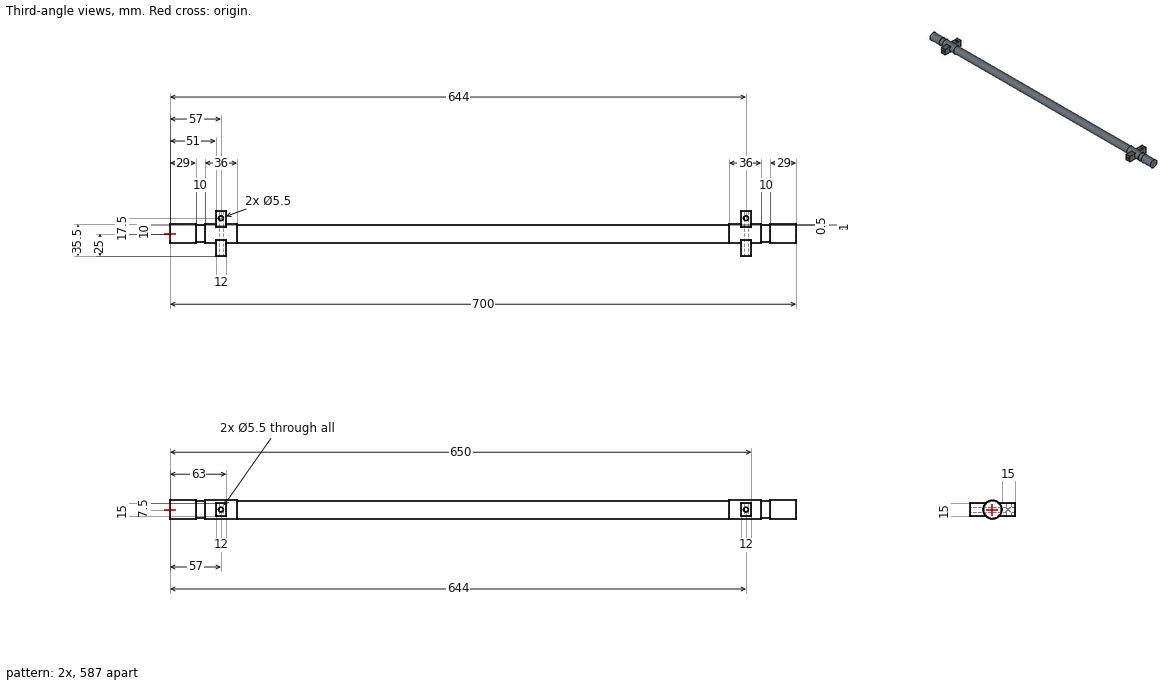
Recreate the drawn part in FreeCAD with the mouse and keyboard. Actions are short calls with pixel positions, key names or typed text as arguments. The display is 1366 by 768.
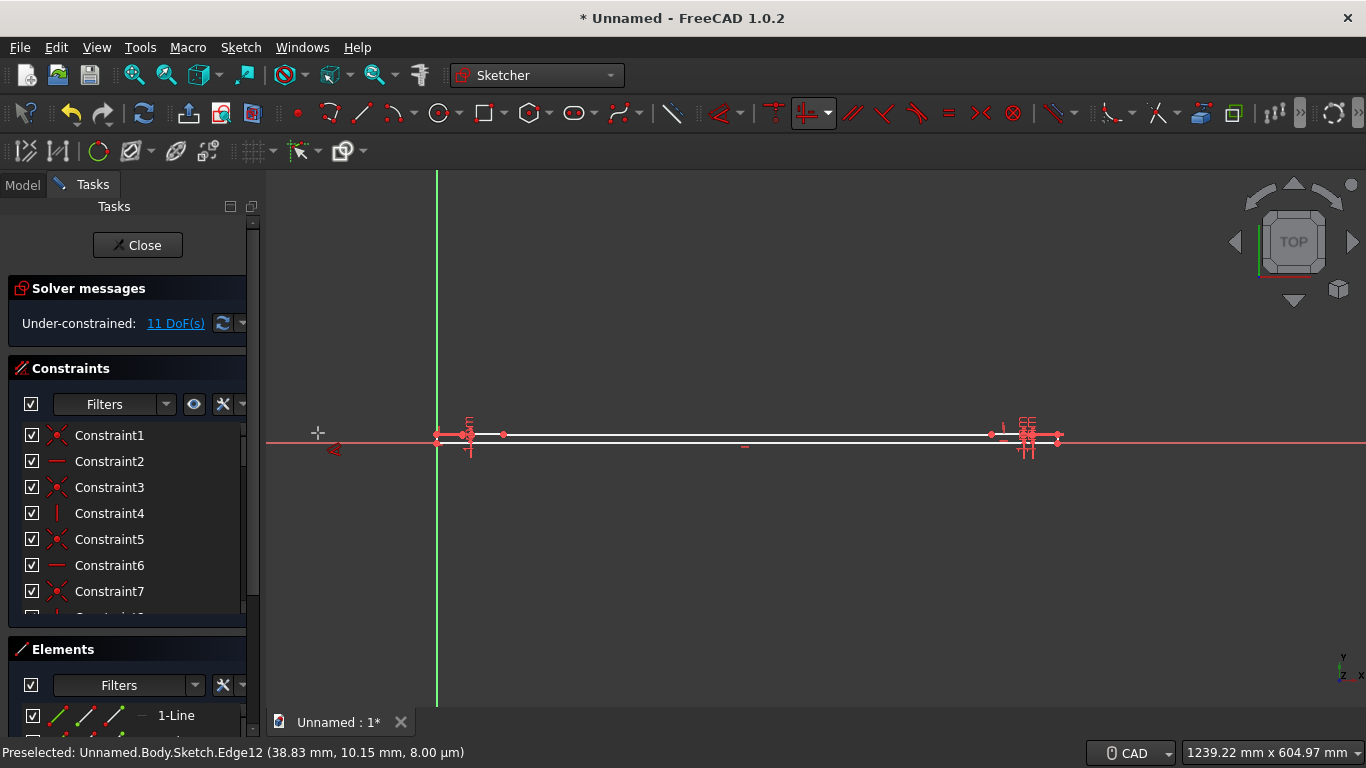
scroll(462, 435, up, 20)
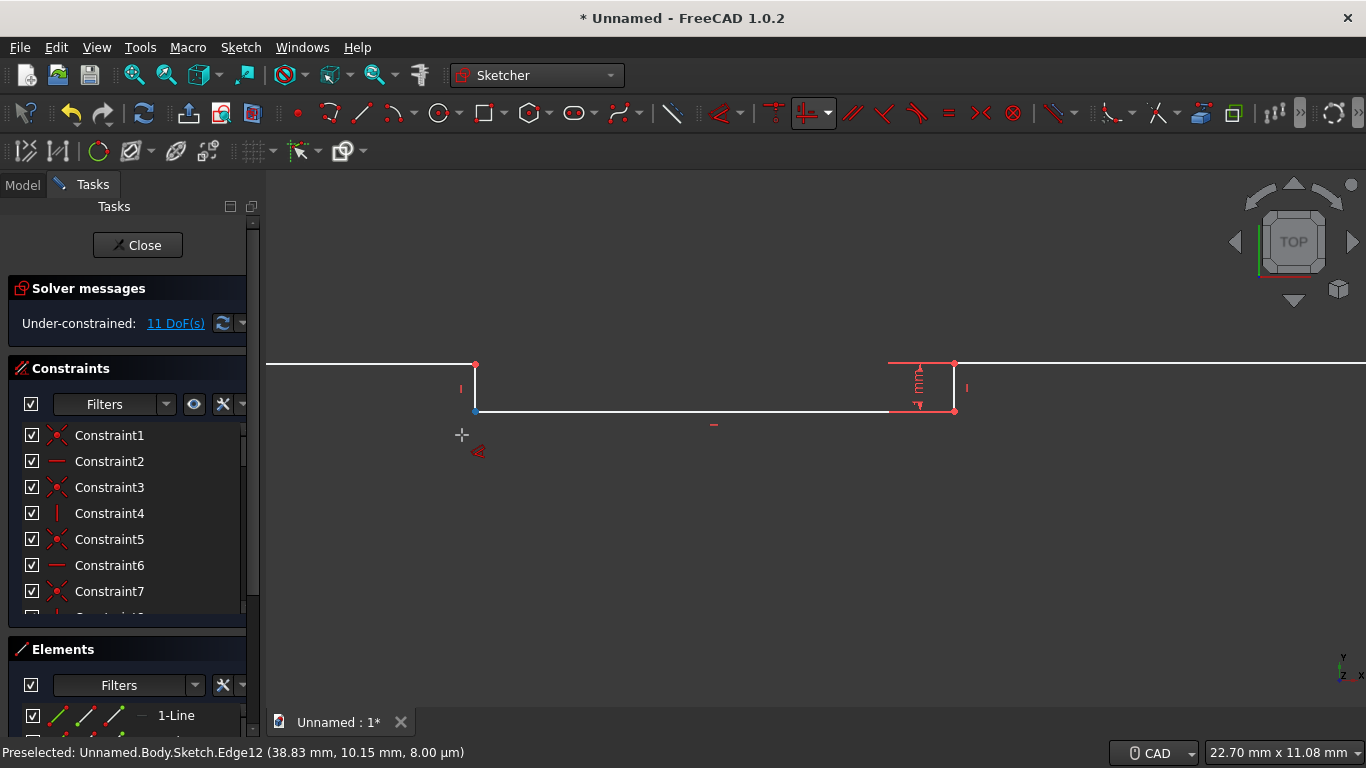
click(475, 397)
click(441, 388)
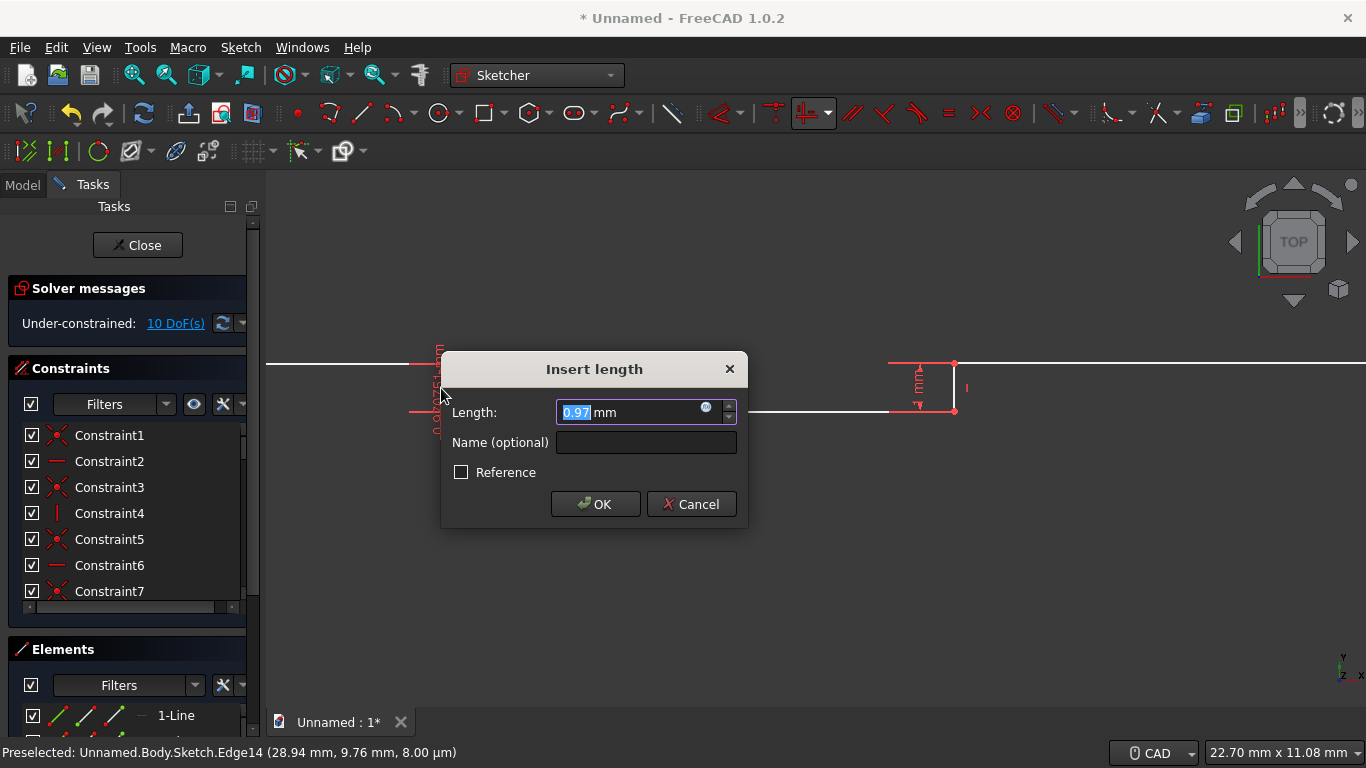
text(1)
key(Return)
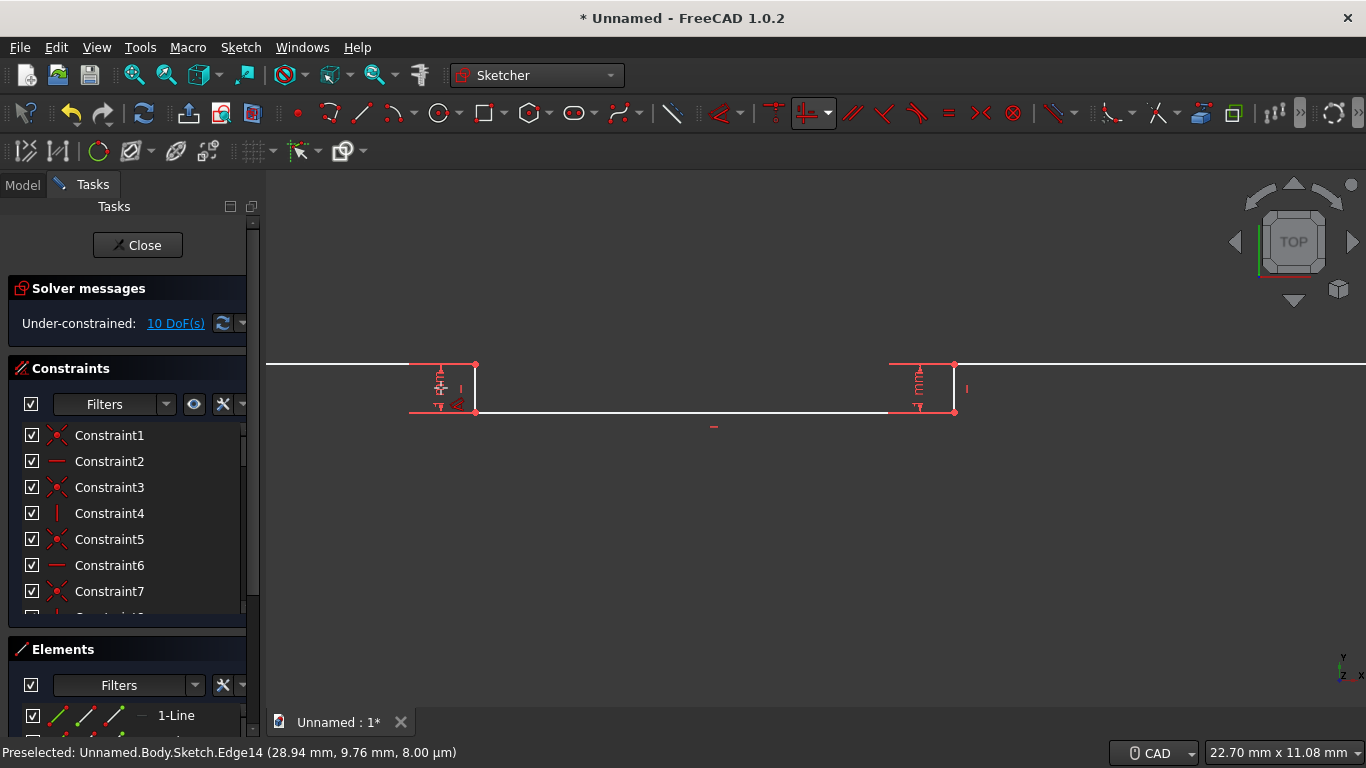
scroll(748, 438, down, 15)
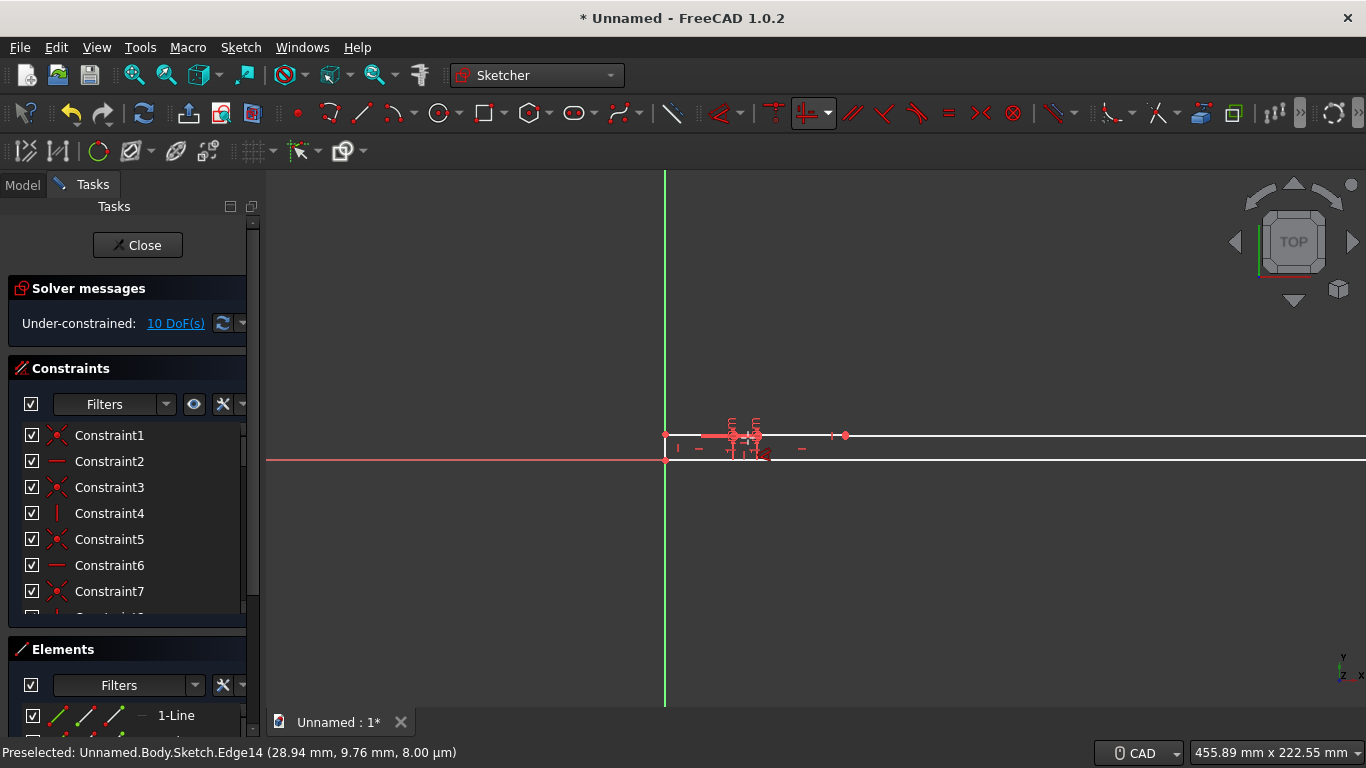
scroll(304, 433, down, 5)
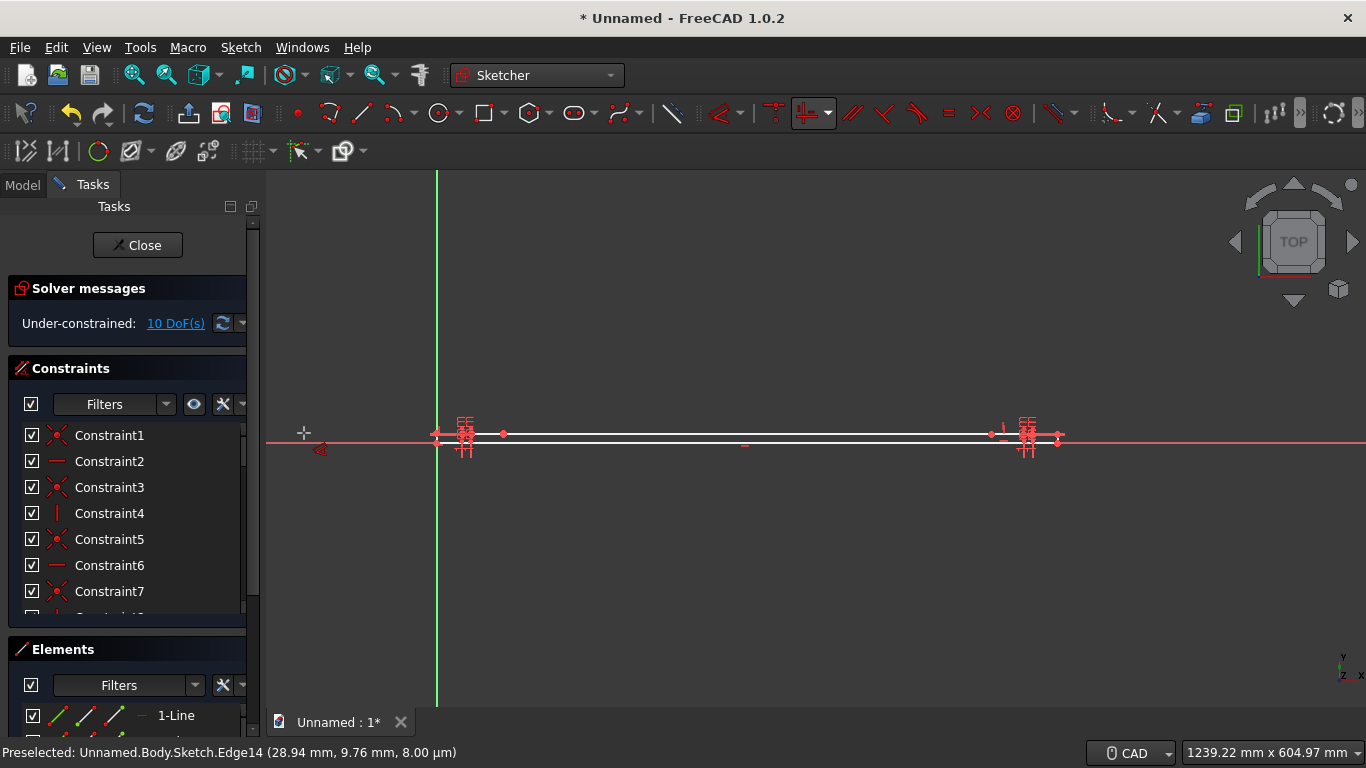
scroll(1050, 434, up, 3)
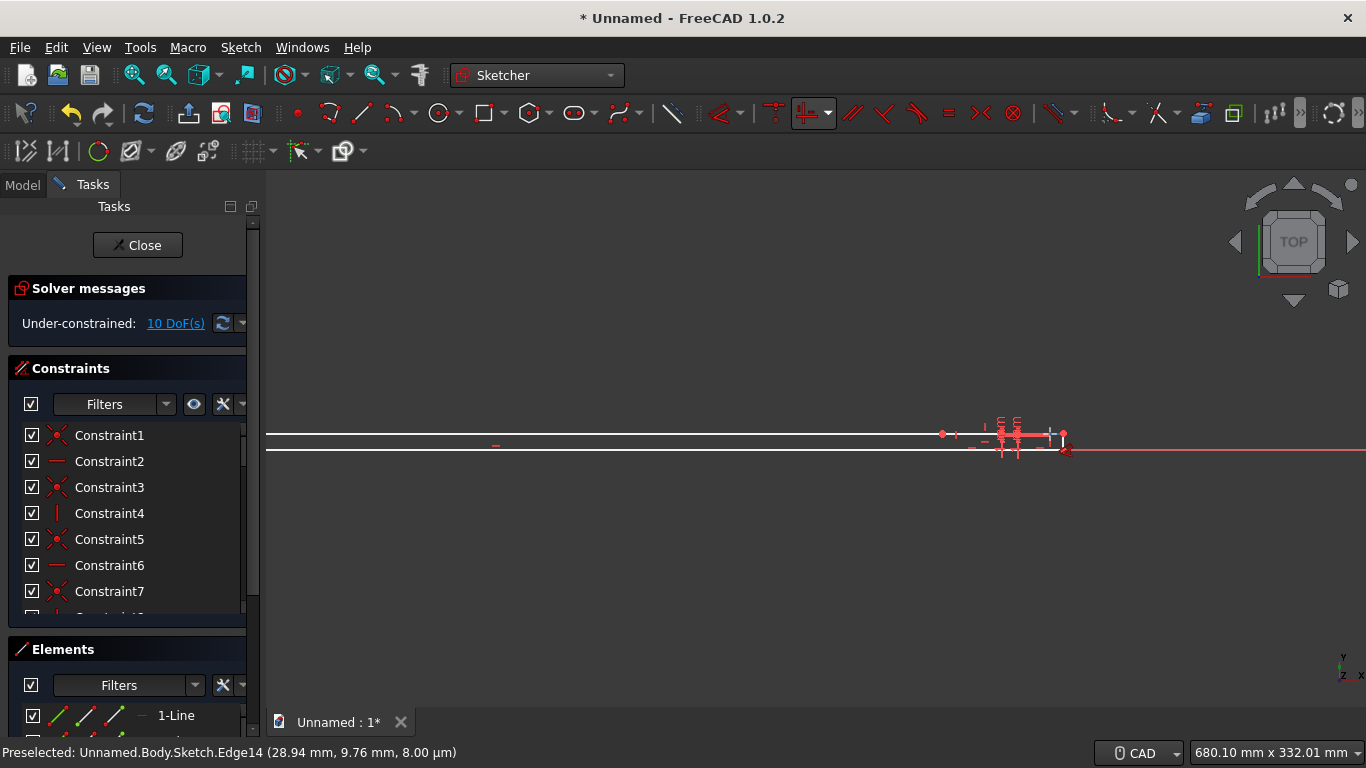
click(1050, 434)
click(1040, 400)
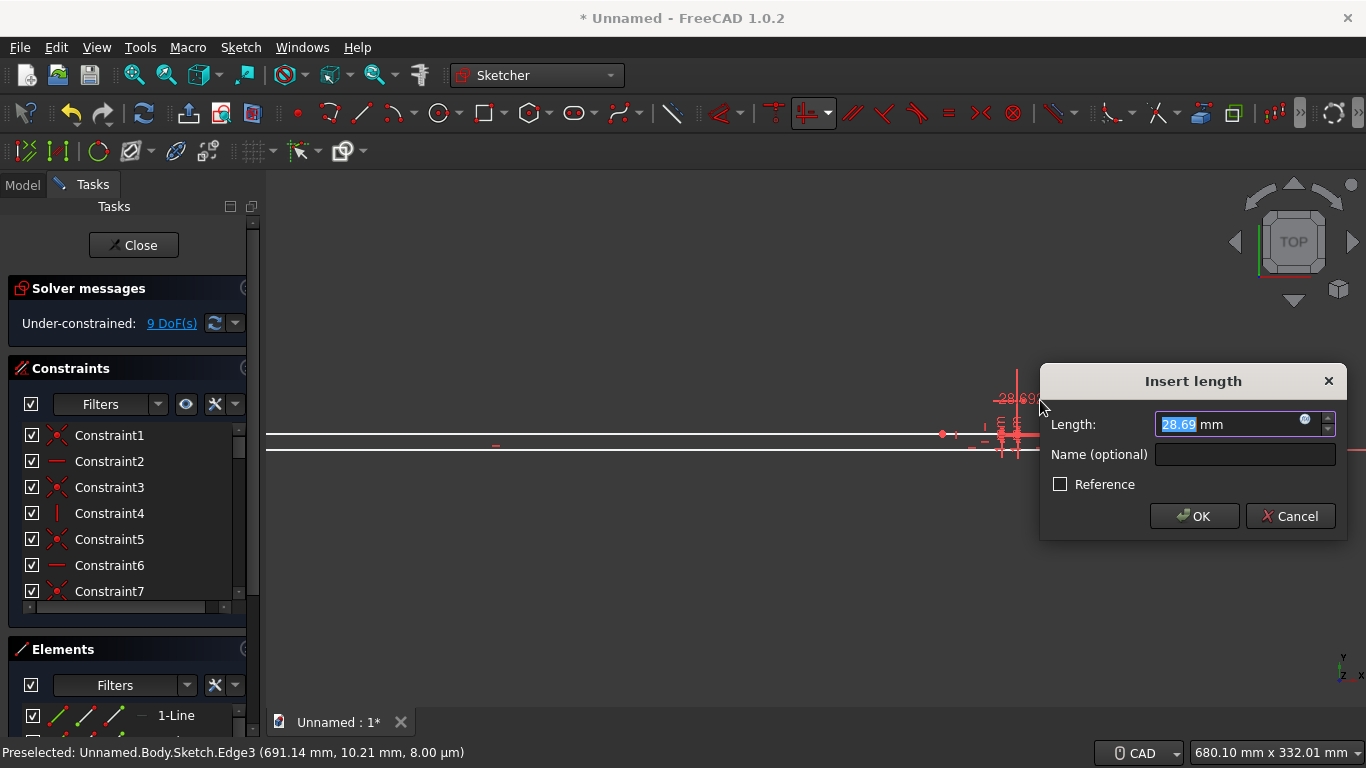
text(29)
key(Return)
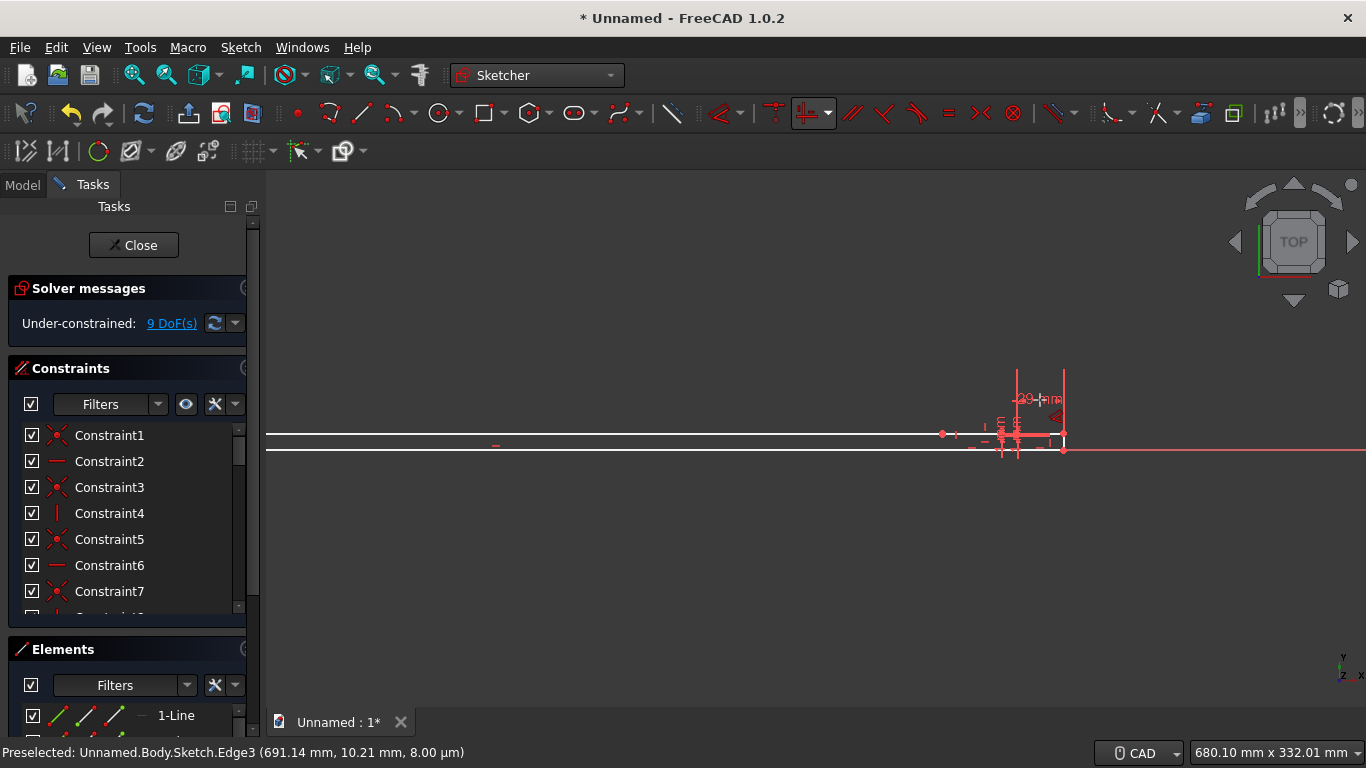
scroll(1009, 436, up, 5)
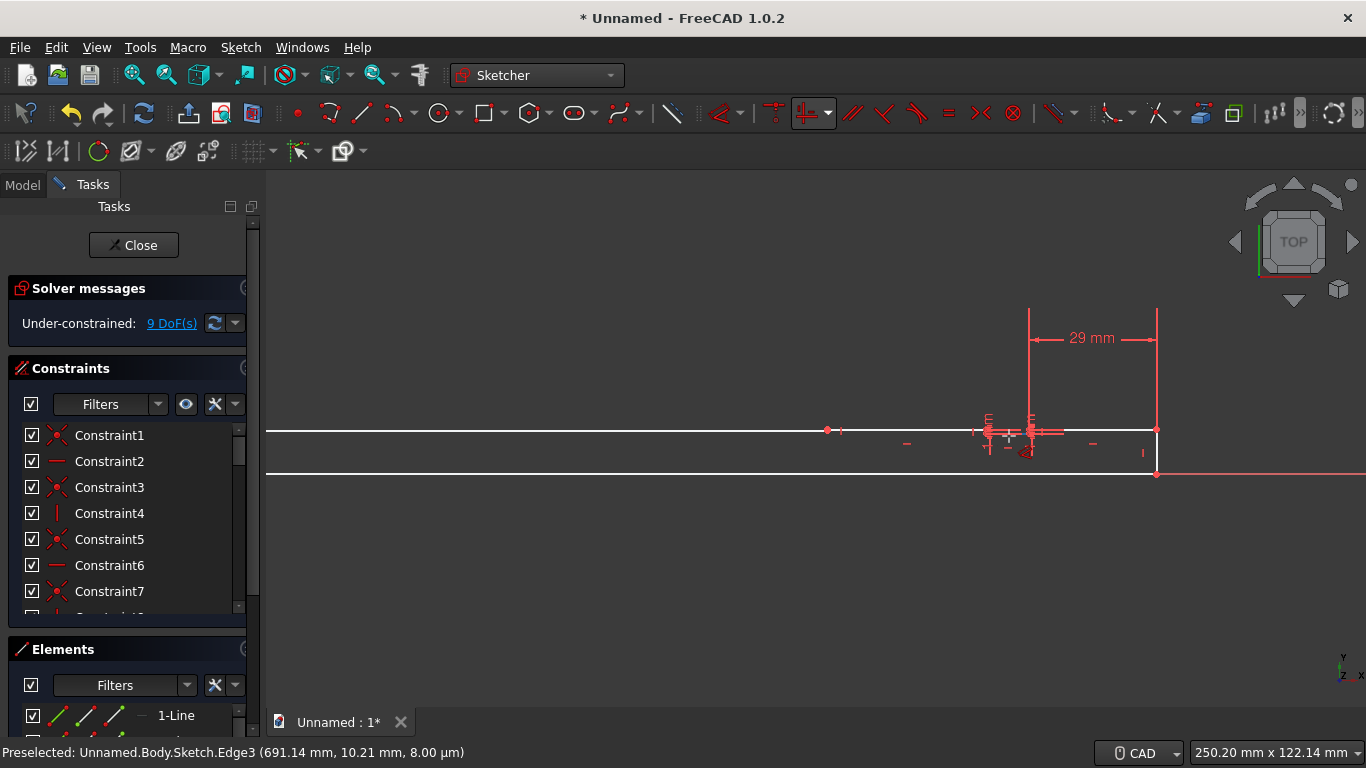
click(1008, 434)
click(1008, 400)